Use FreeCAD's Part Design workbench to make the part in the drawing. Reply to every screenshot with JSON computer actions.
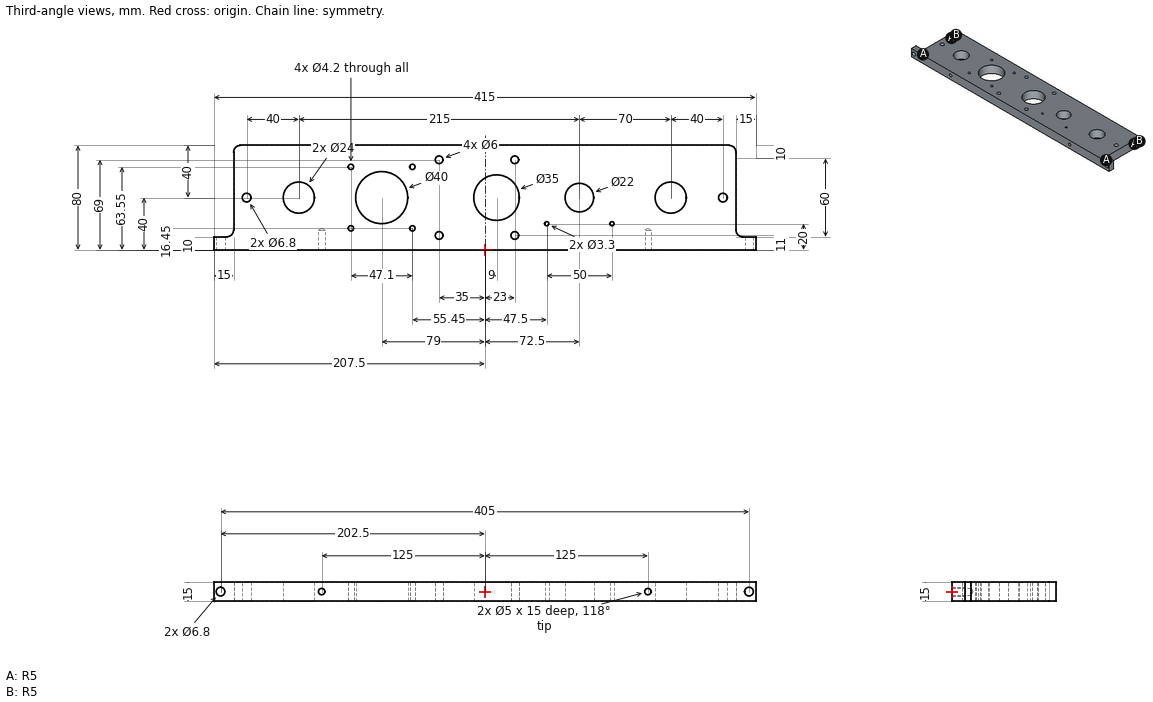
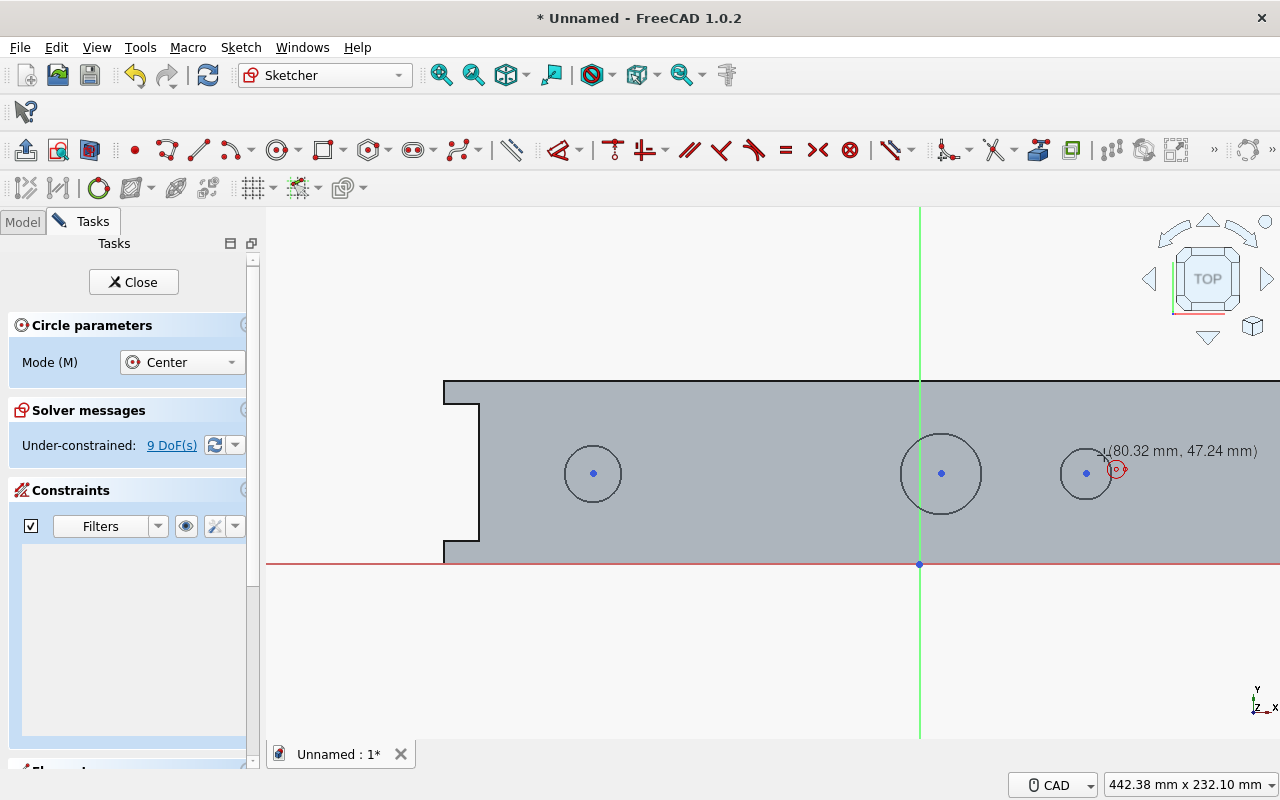
{"action": "left_click", "coordinate": [739, 473]}
{"action": "left_click", "coordinate": [771, 440]}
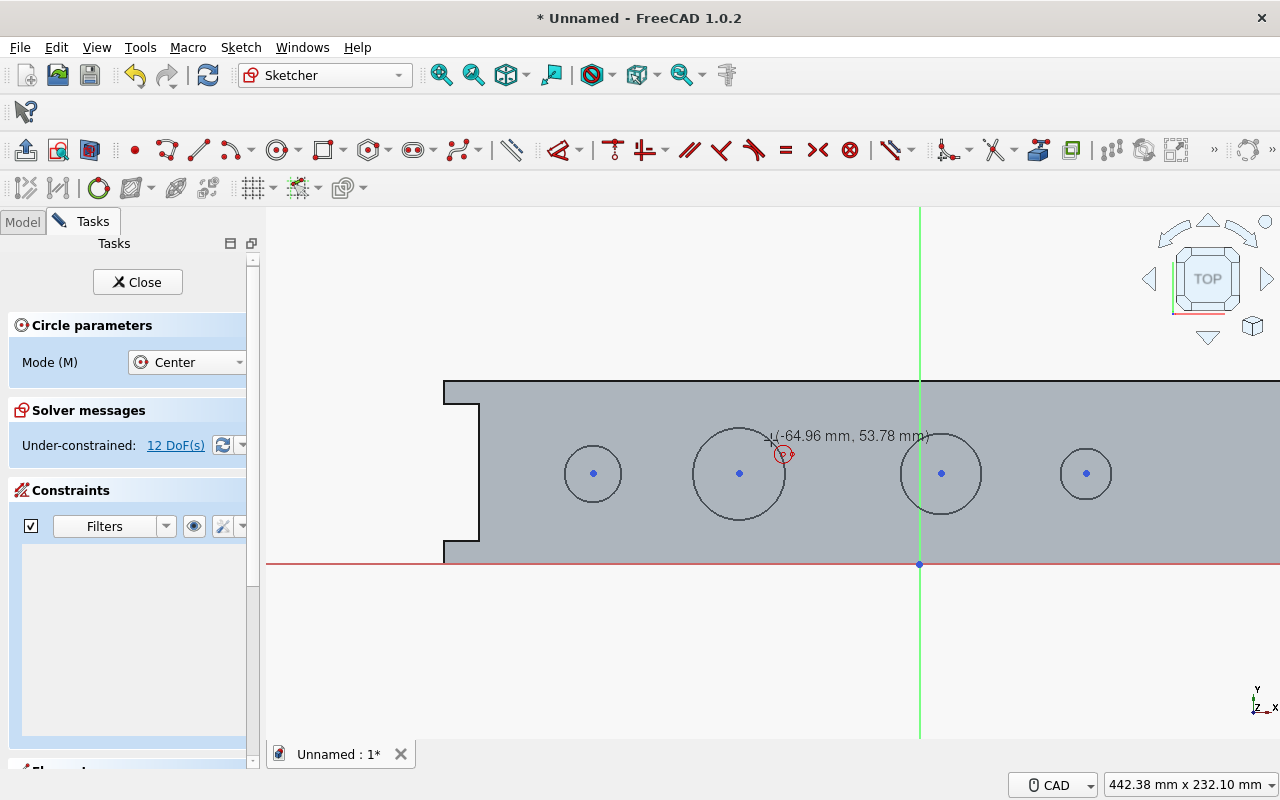
{"action": "scroll", "coordinate": [294, 427], "scroll_direction": "down", "scroll_amount": 2}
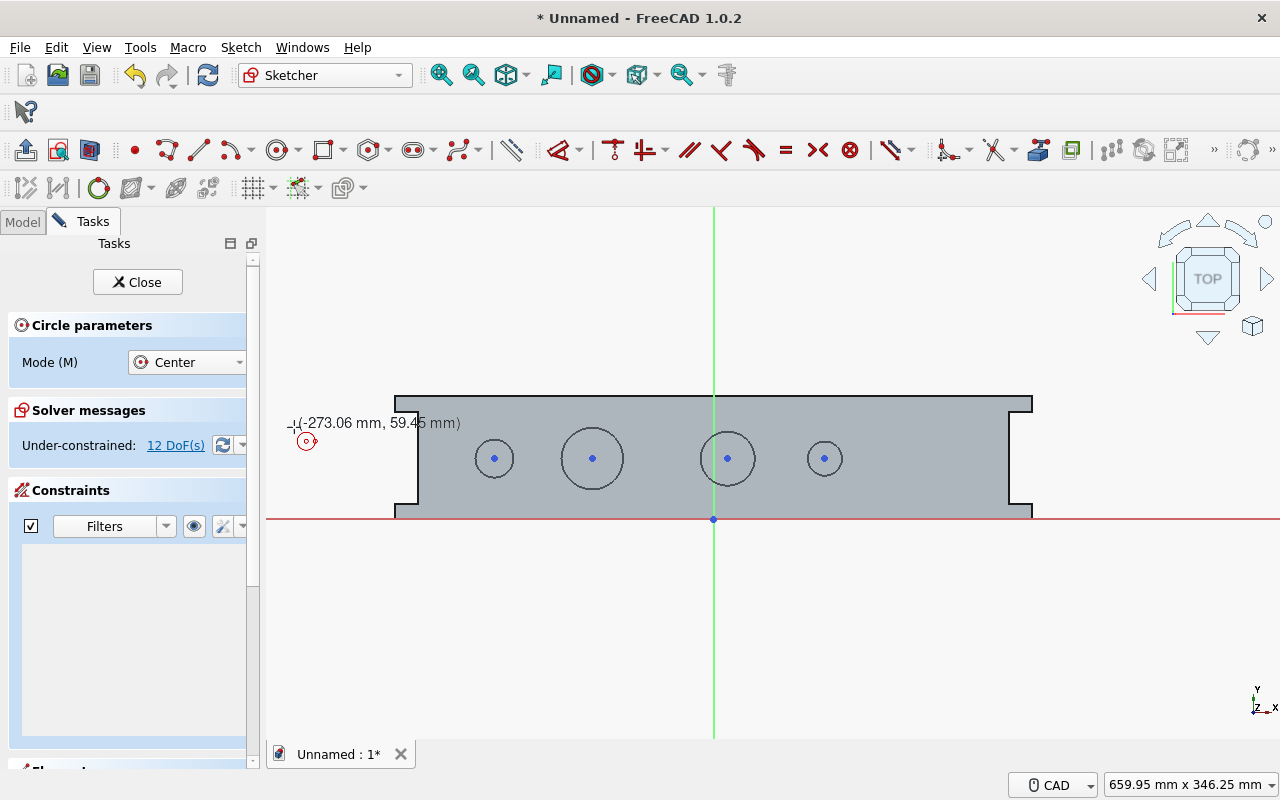
{"action": "scroll", "coordinate": [933, 458], "scroll_direction": "up", "scroll_amount": 2}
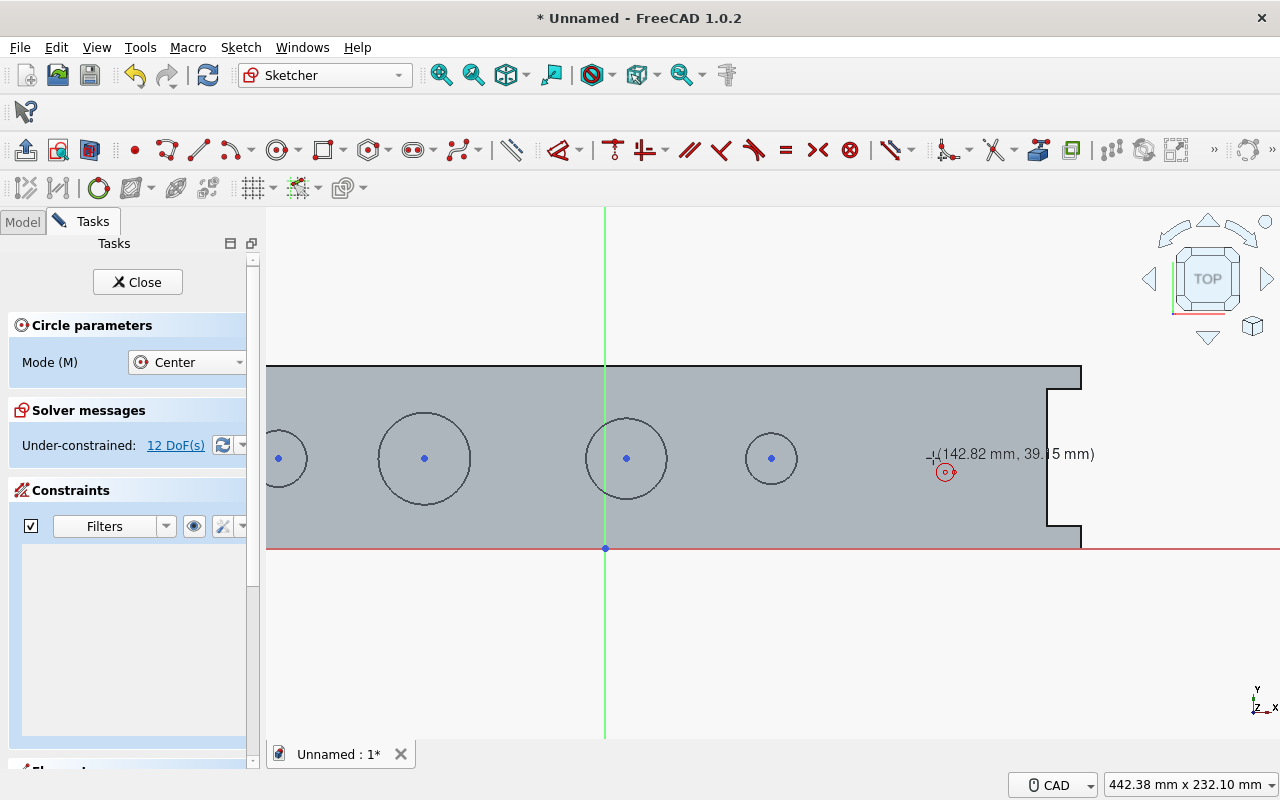
{"action": "left_click", "coordinate": [932, 457]}
{"action": "left_click", "coordinate": [951, 438]}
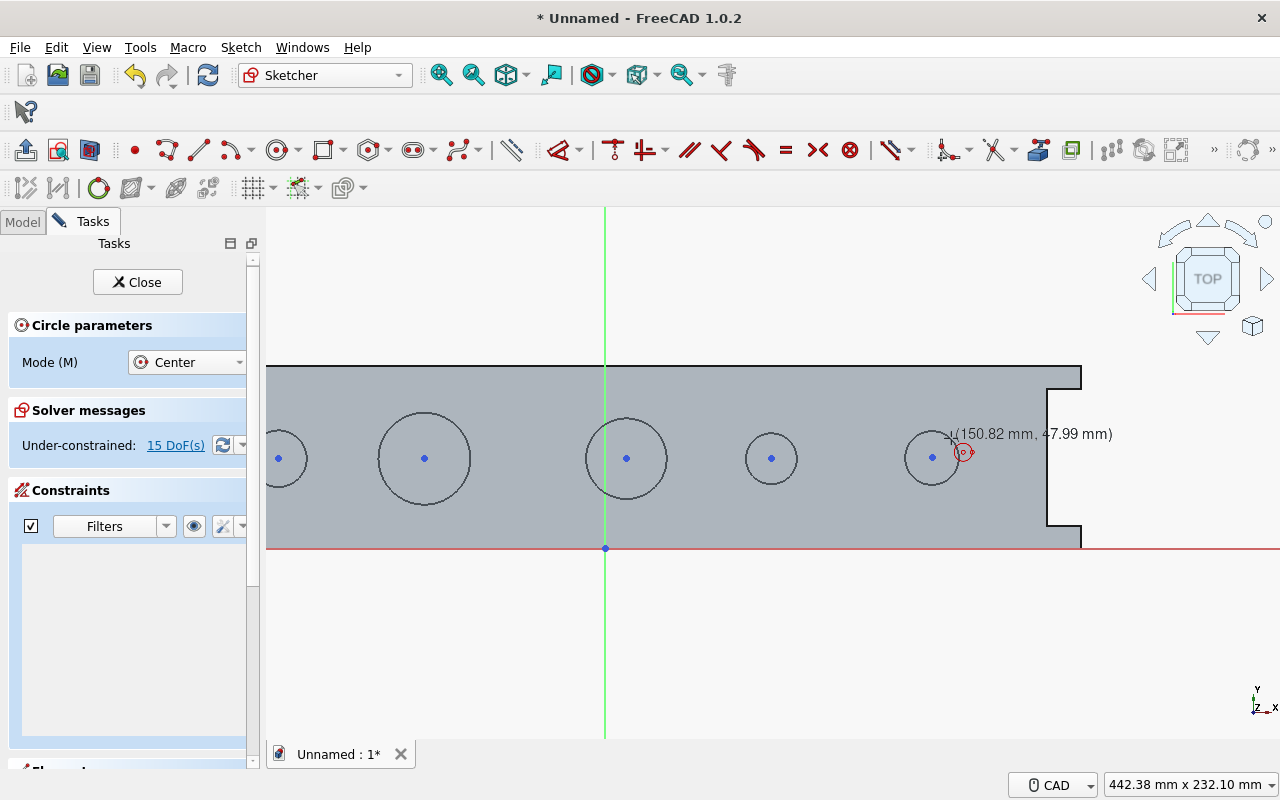
{"action": "scroll", "coordinate": [906, 458], "scroll_direction": "down", "scroll_amount": 2}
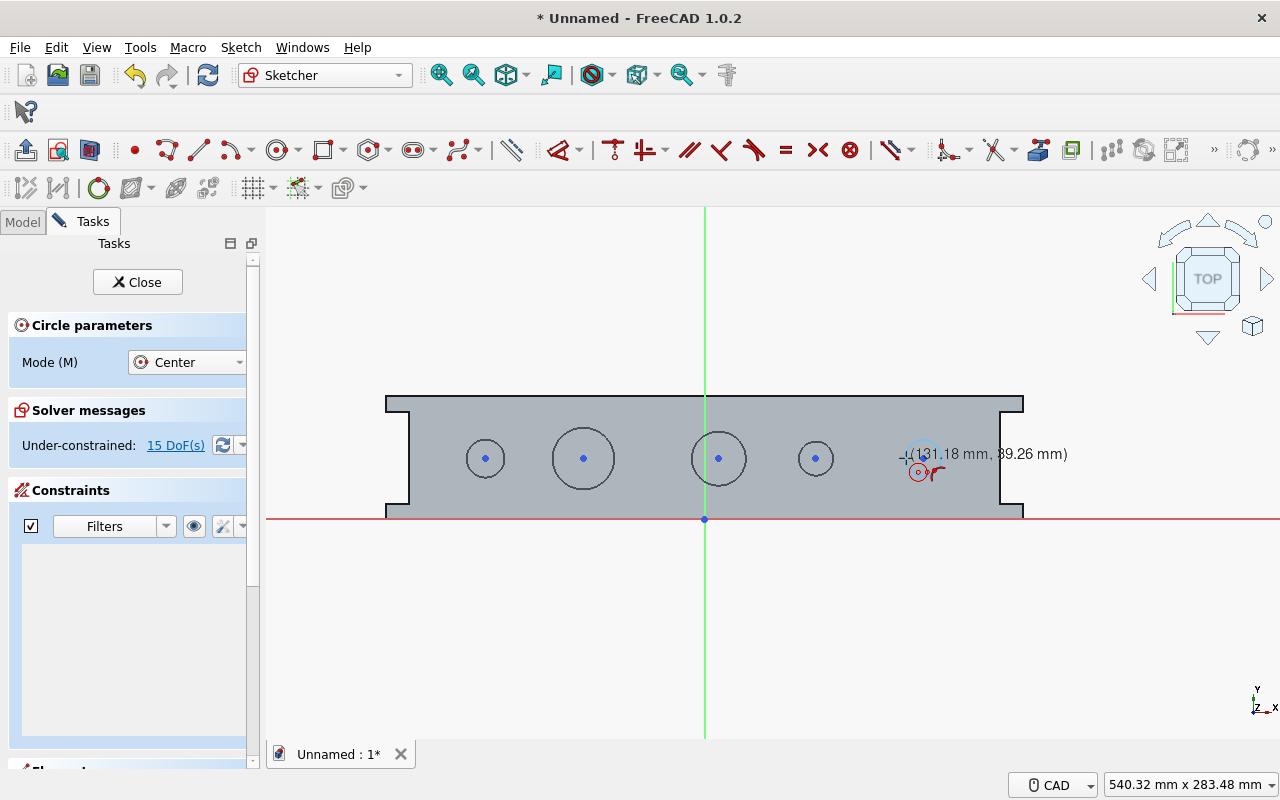
{"action": "scroll", "coordinate": [424, 458], "scroll_direction": "up", "scroll_amount": 8}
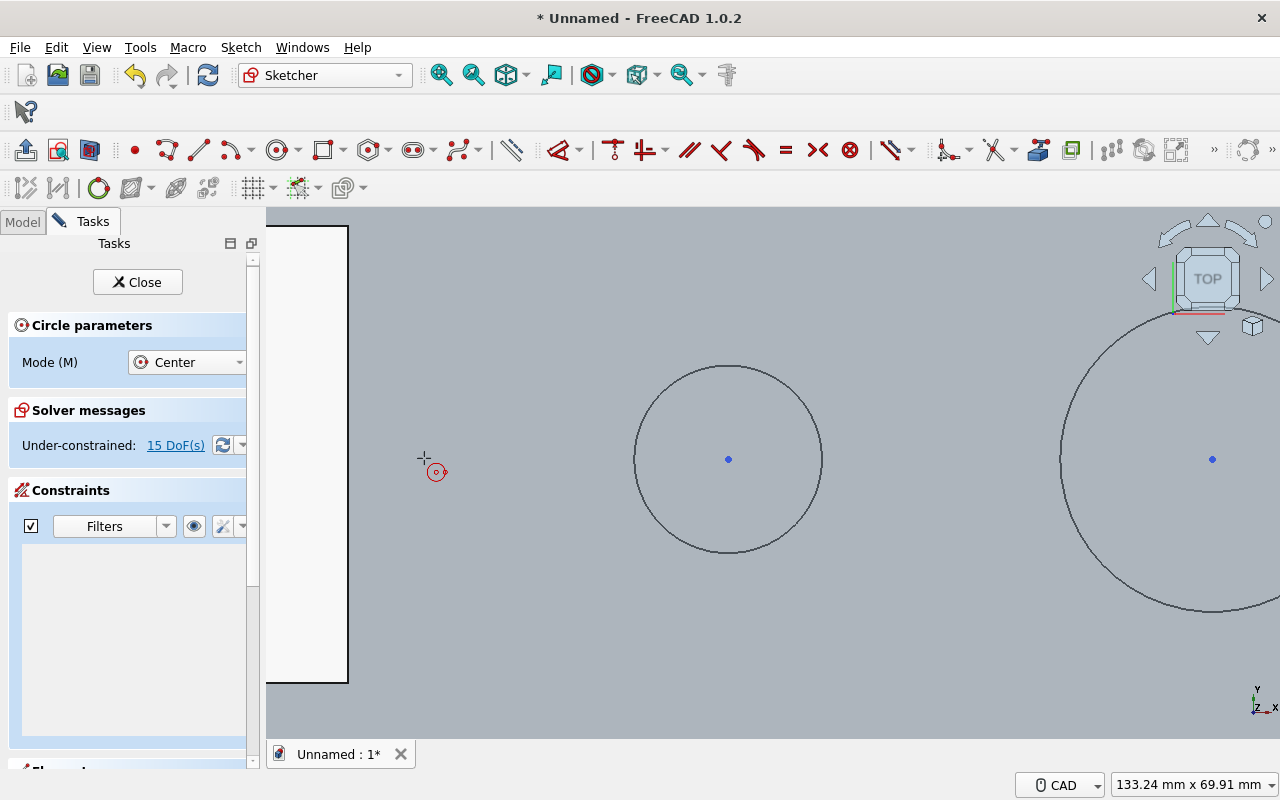
{"action": "scroll", "coordinate": [424, 458], "scroll_direction": "down", "scroll_amount": 8}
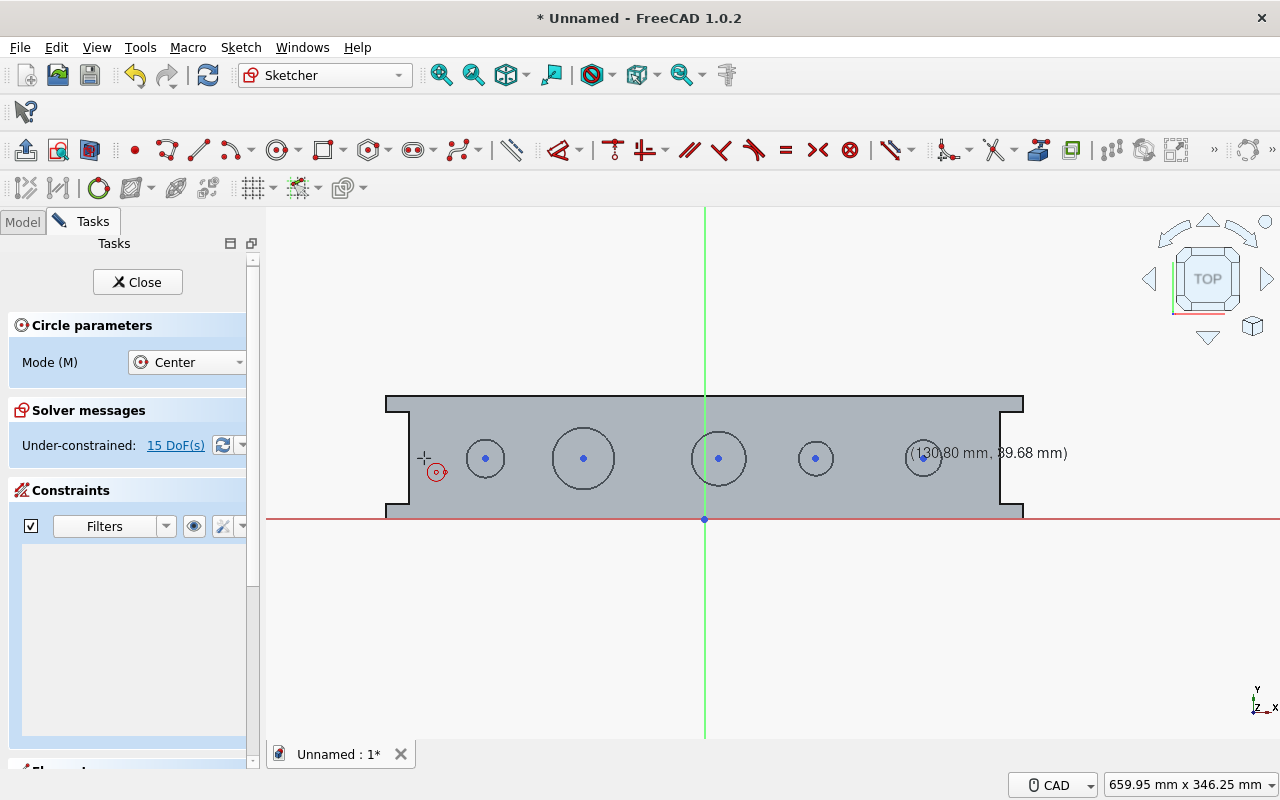
{"action": "left_click", "coordinate": [424, 458]}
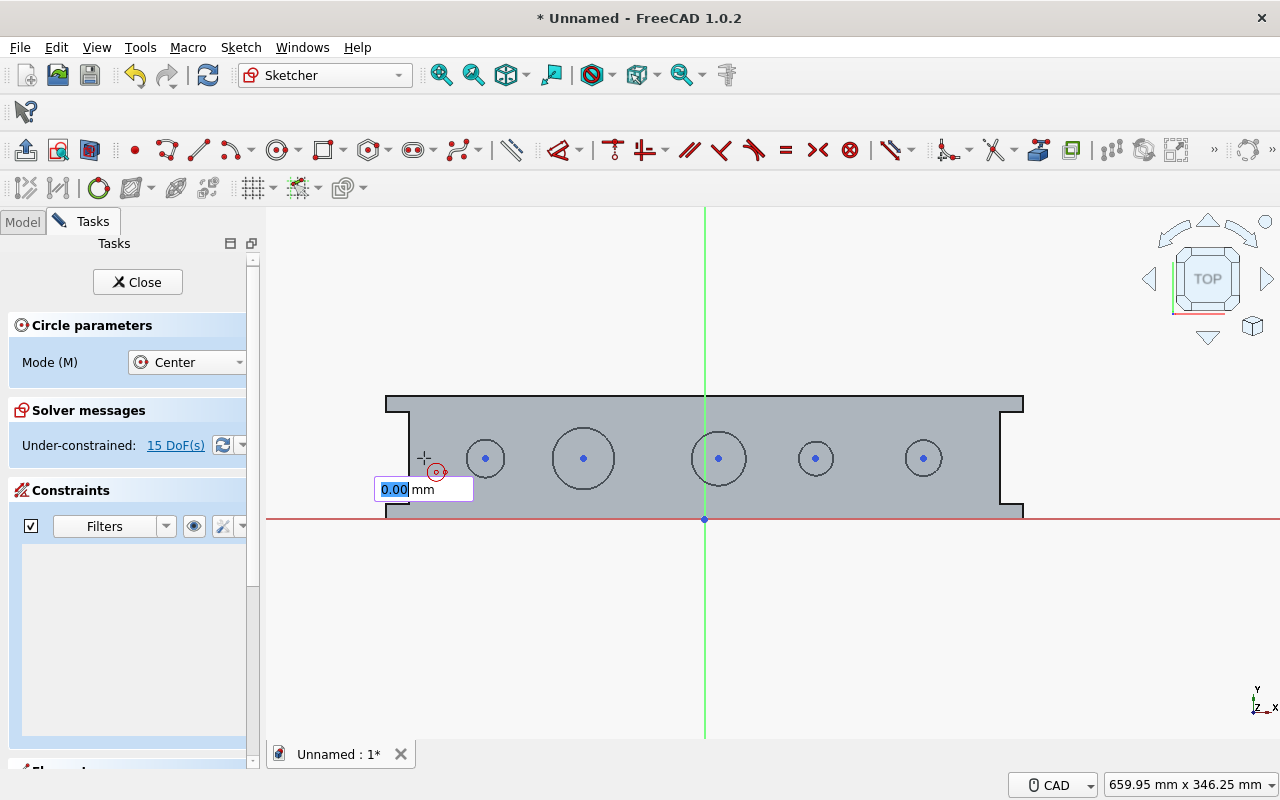
{"action": "scroll", "coordinate": [428, 454], "scroll_direction": "up", "scroll_amount": 6}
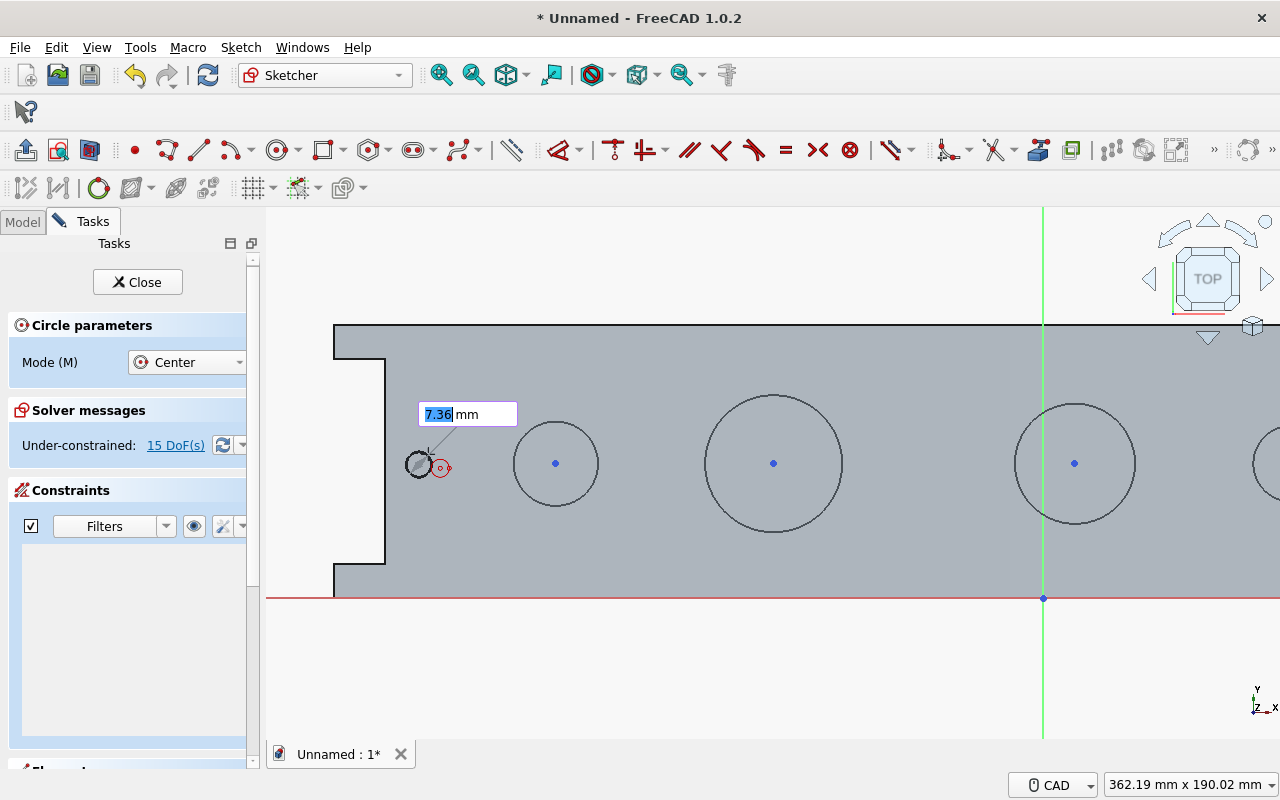
{"action": "left_click", "coordinate": [427, 453]}